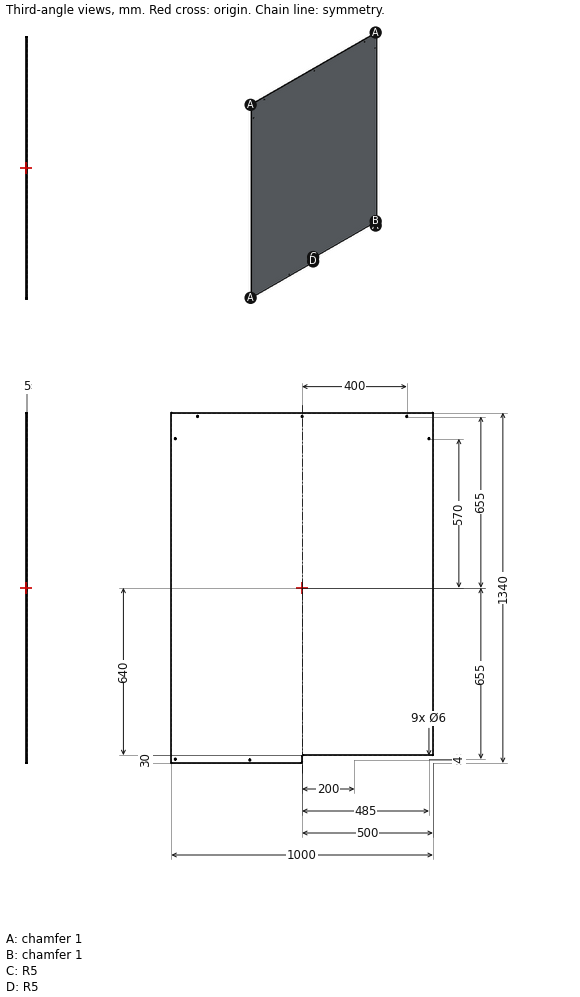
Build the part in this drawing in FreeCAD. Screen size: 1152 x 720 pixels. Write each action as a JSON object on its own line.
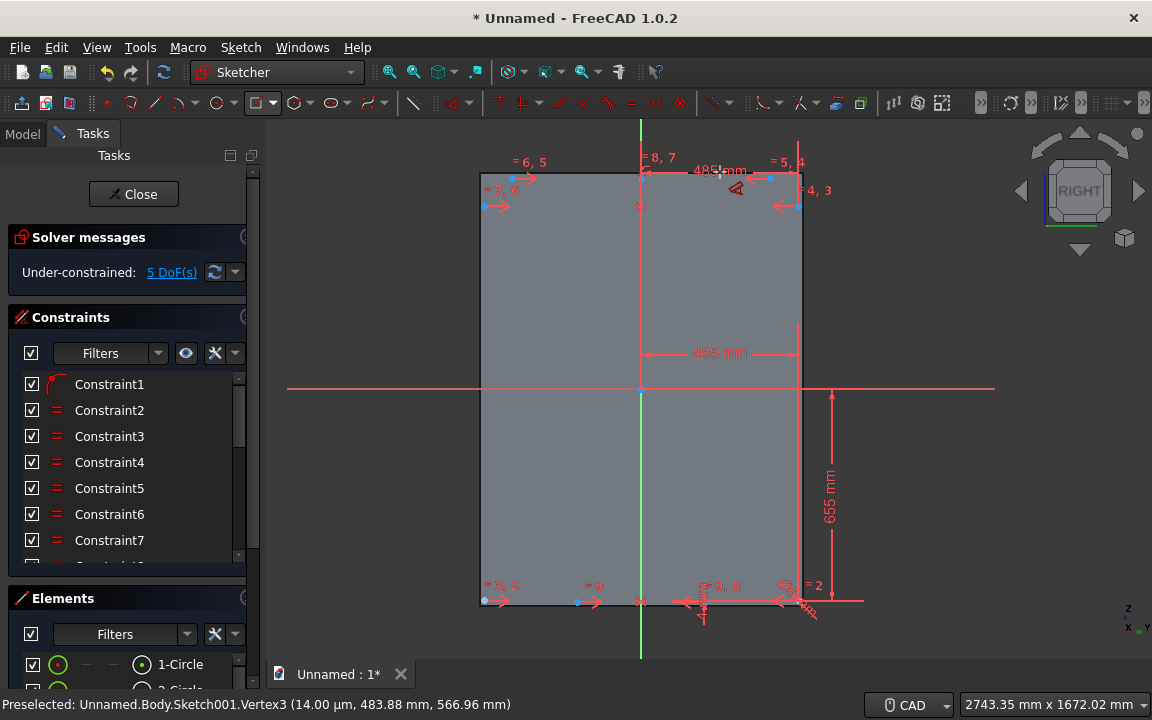
{"action": "left_click", "coordinate": [798, 206]}
{"action": "left_click", "coordinate": [832, 298]}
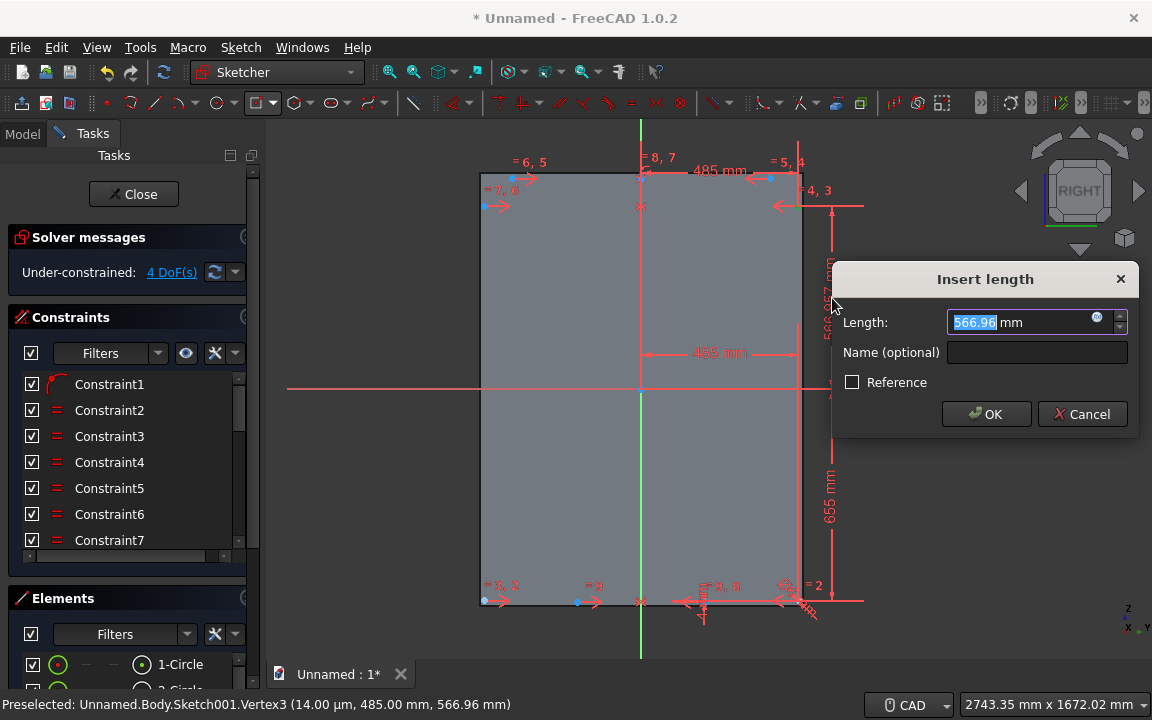
{"action": "type", "text": "570"}
{"action": "key", "text": "Return"}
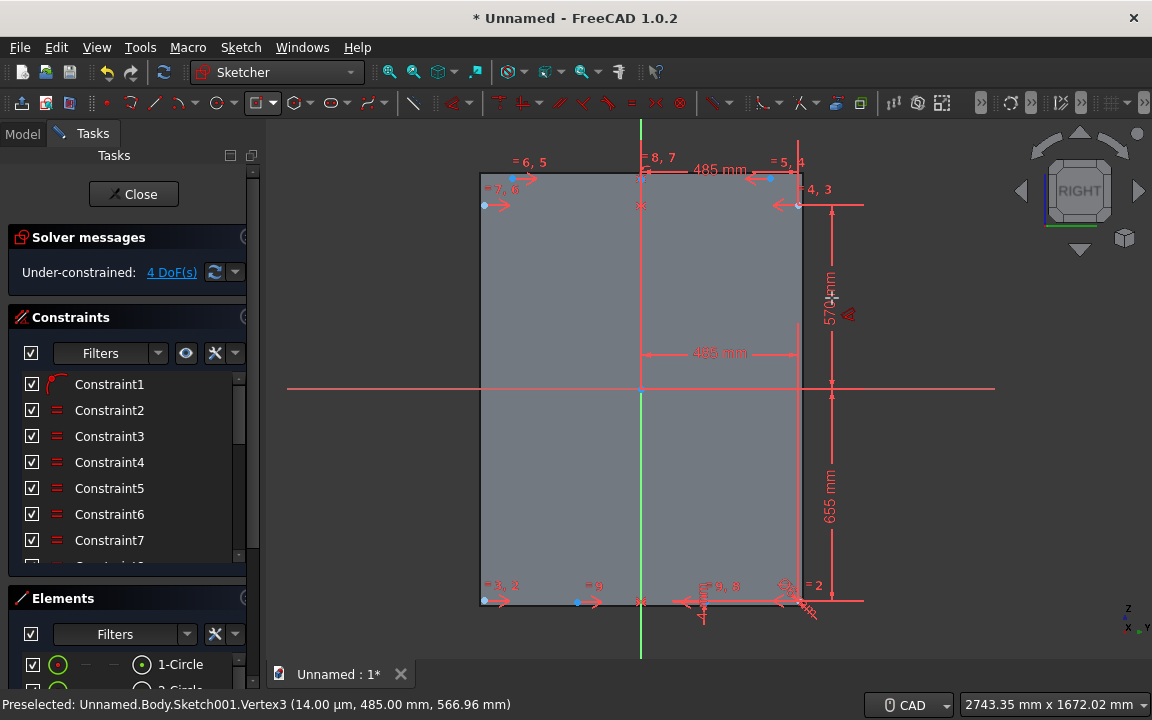
{"action": "left_click", "coordinate": [771, 179]}
{"action": "left_click", "coordinate": [706, 423]}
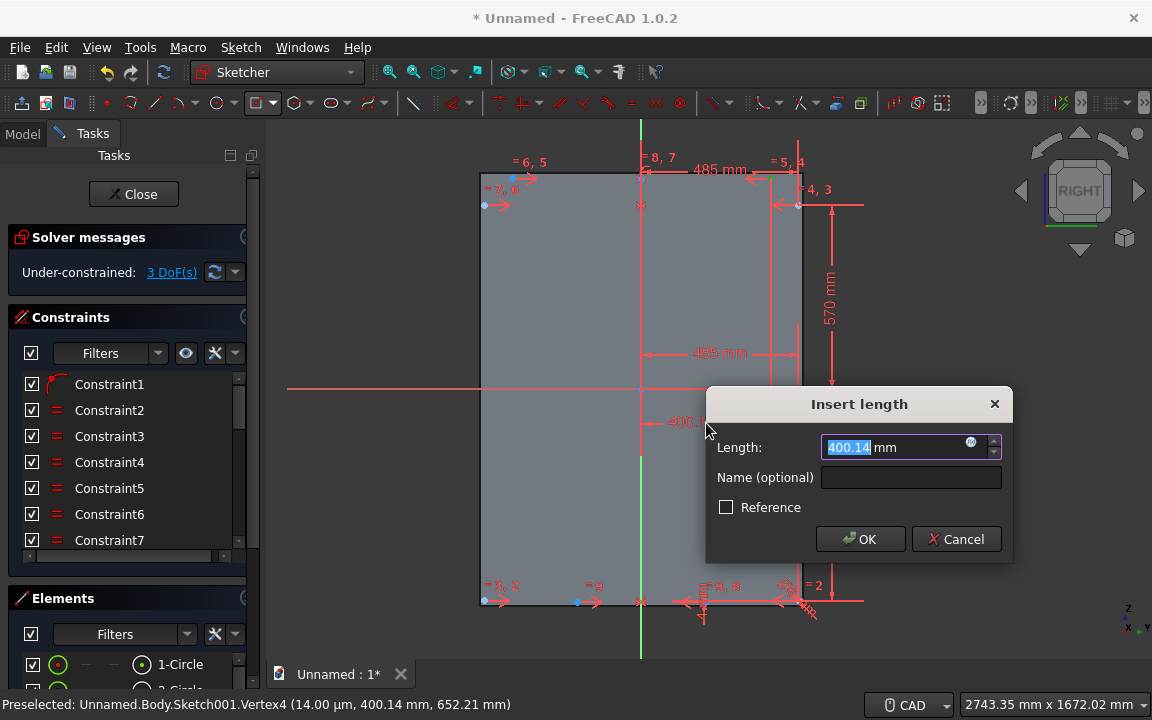
{"action": "type", "text": "400"}
{"action": "key", "text": "Return"}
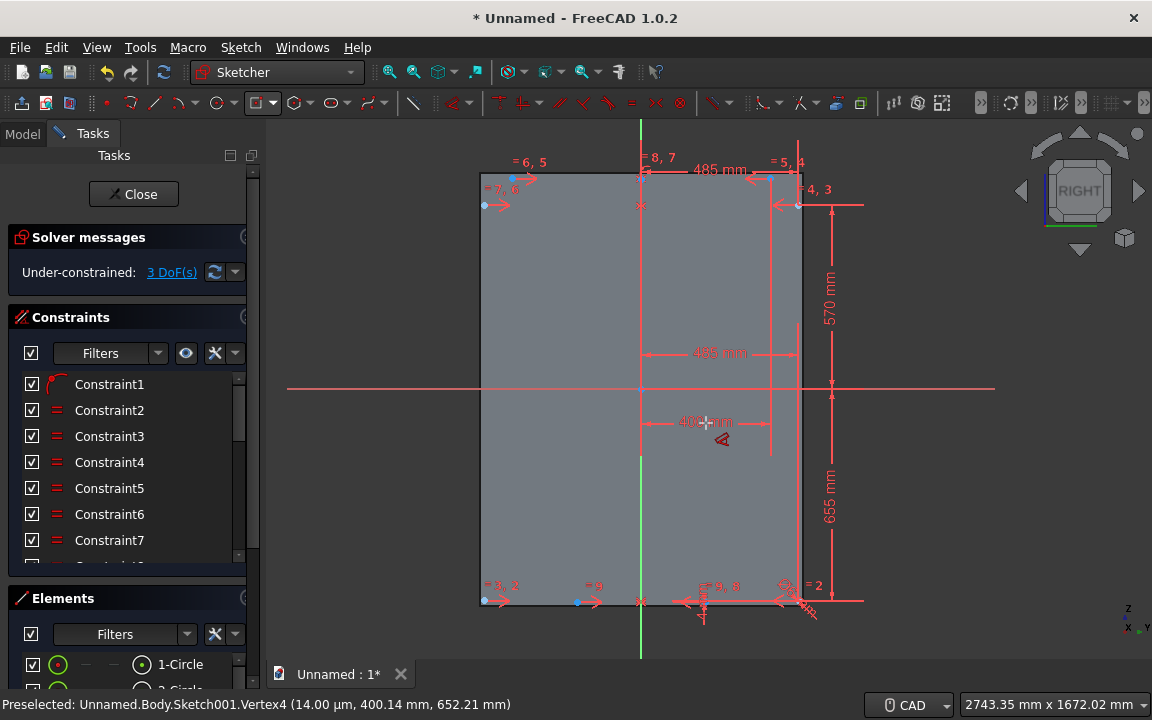
{"action": "left_click", "coordinate": [771, 179]}
{"action": "left_click", "coordinate": [805, 236]}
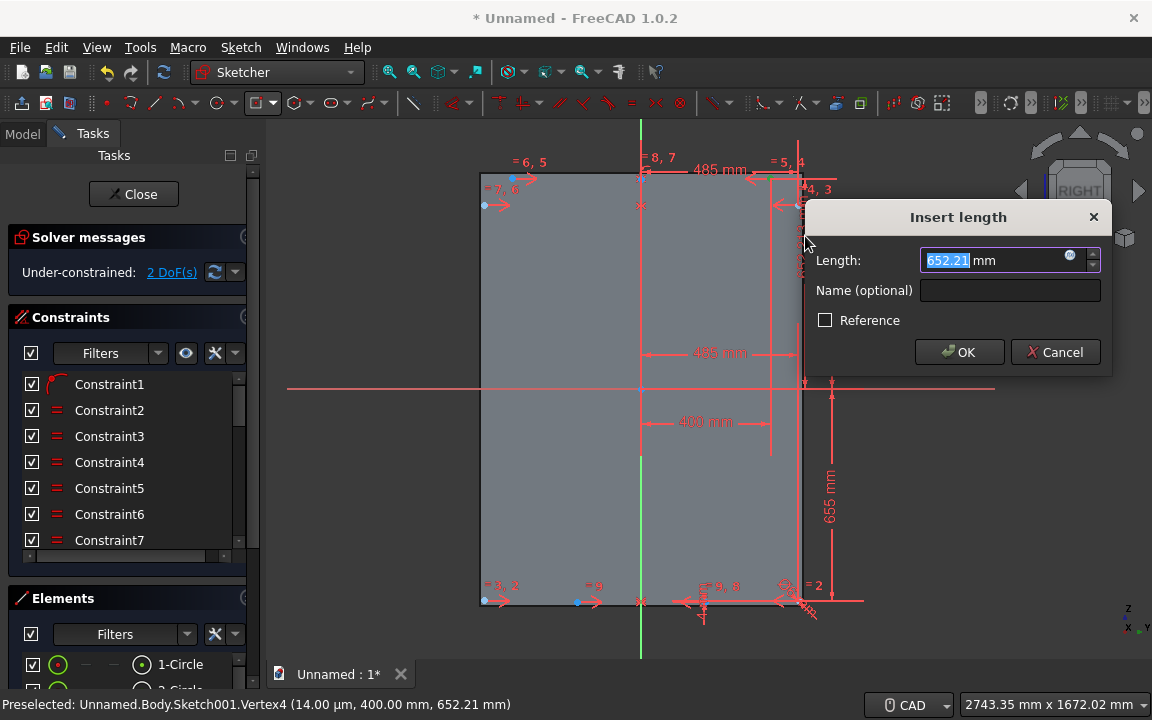
{"action": "type", "text": "655"}
{"action": "key", "text": "Return"}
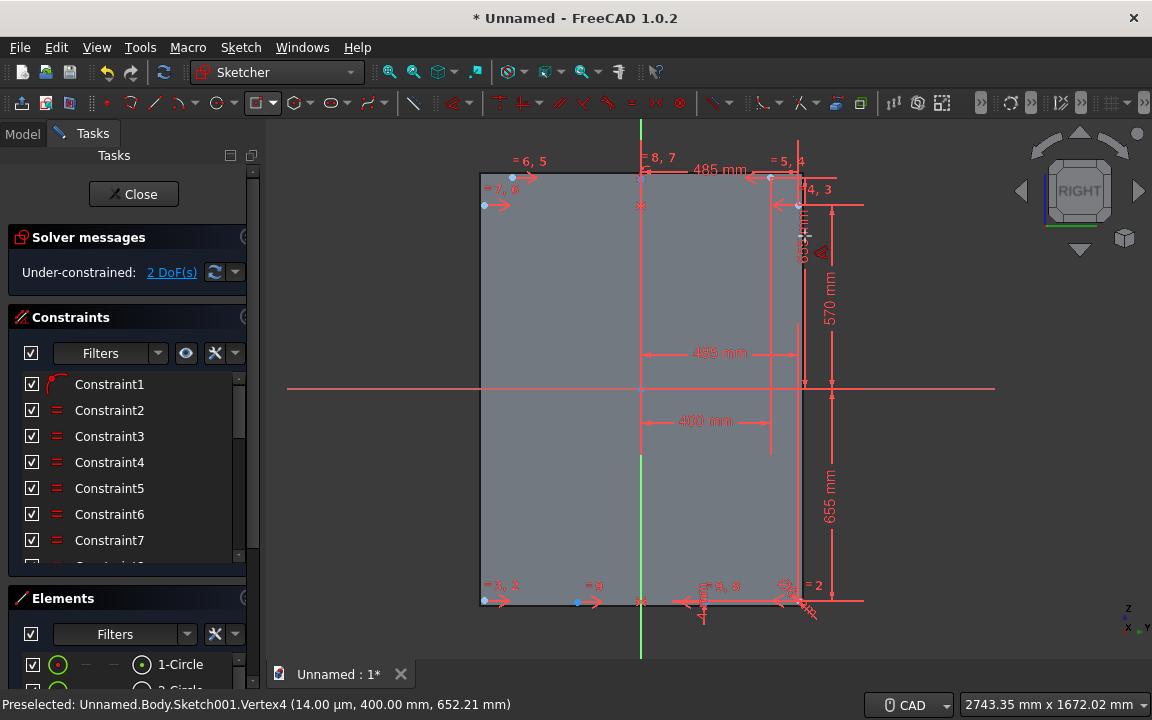
{"action": "left_click", "coordinate": [641, 179]}
{"action": "left_click", "coordinate": [675, 284]}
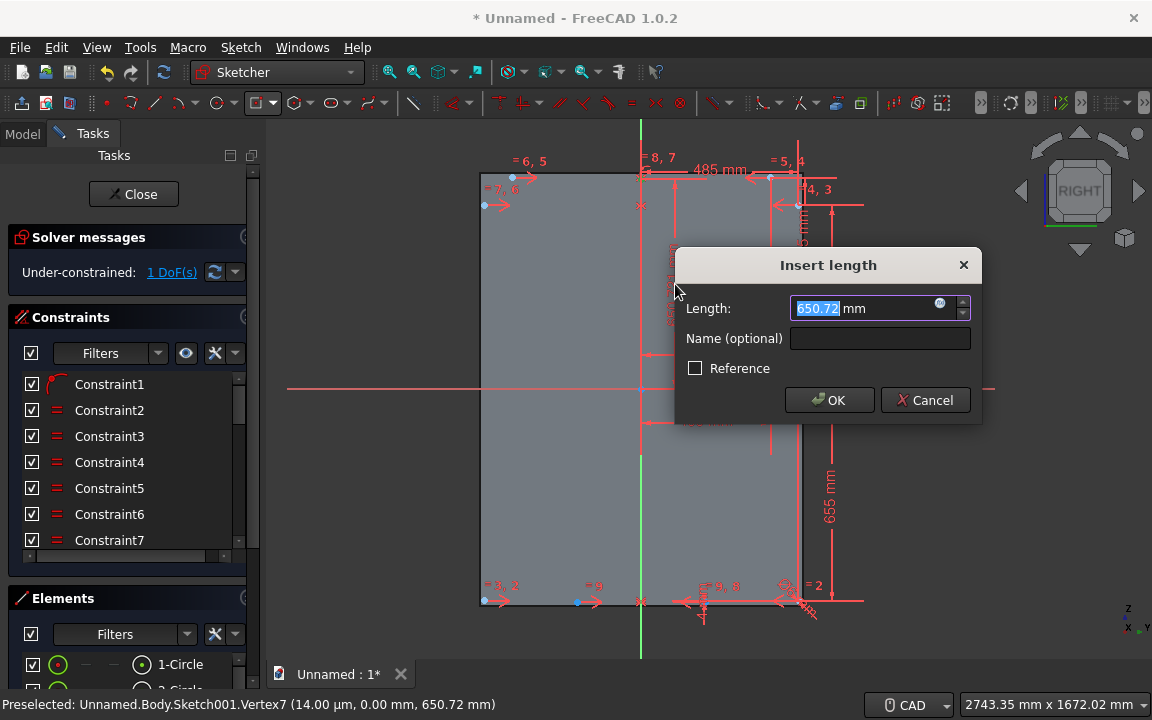
{"action": "type", "text": "655"}
{"action": "key", "text": "Return"}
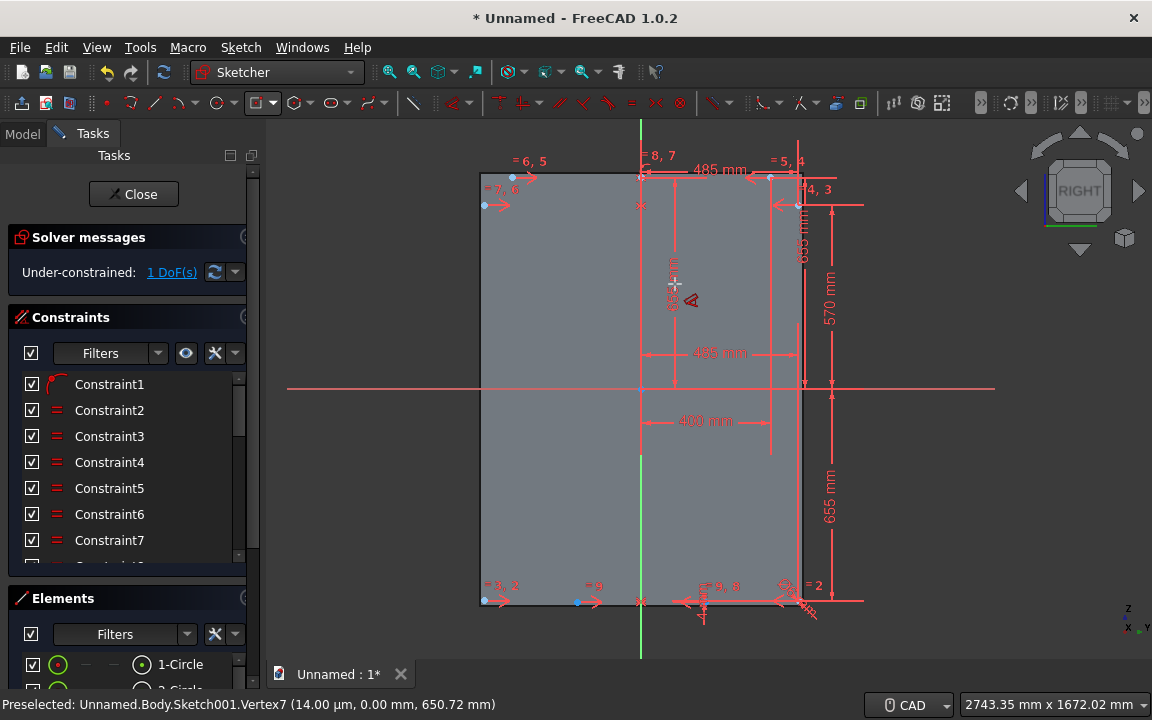
{"action": "left_click", "coordinate": [706, 602]}
{"action": "left_click", "coordinate": [674, 331]}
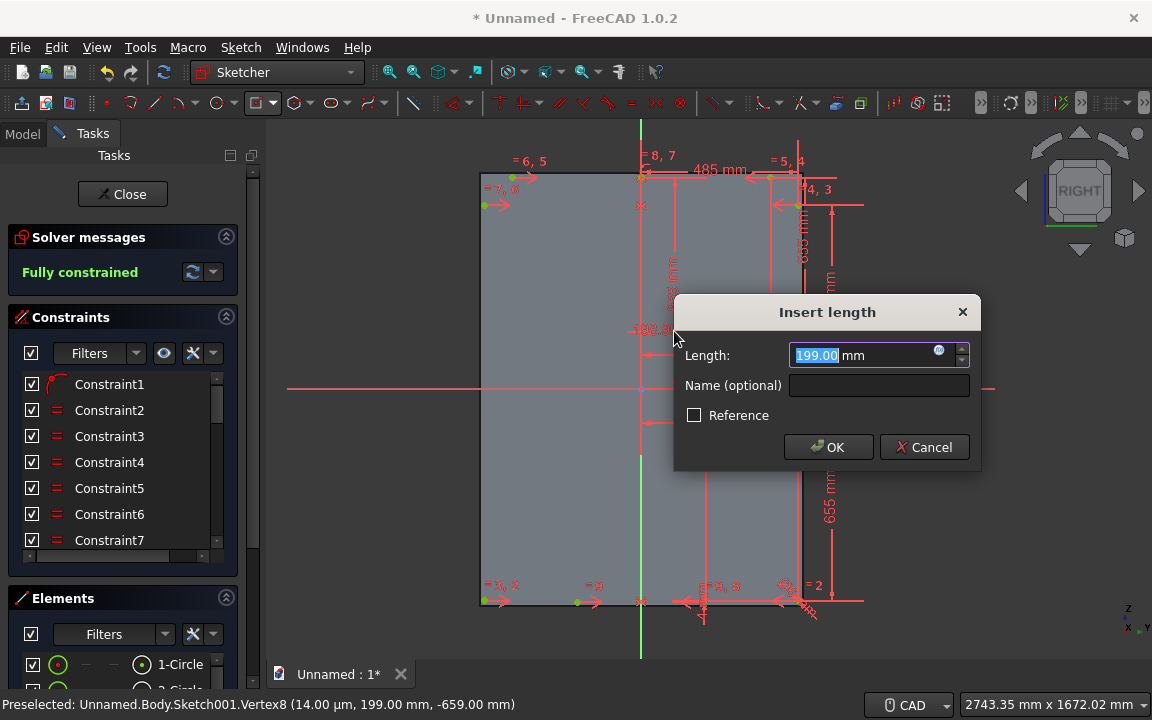
{"action": "type", "text": "200"}
{"action": "key", "text": "Return"}
{"action": "key", "text": "Escape"}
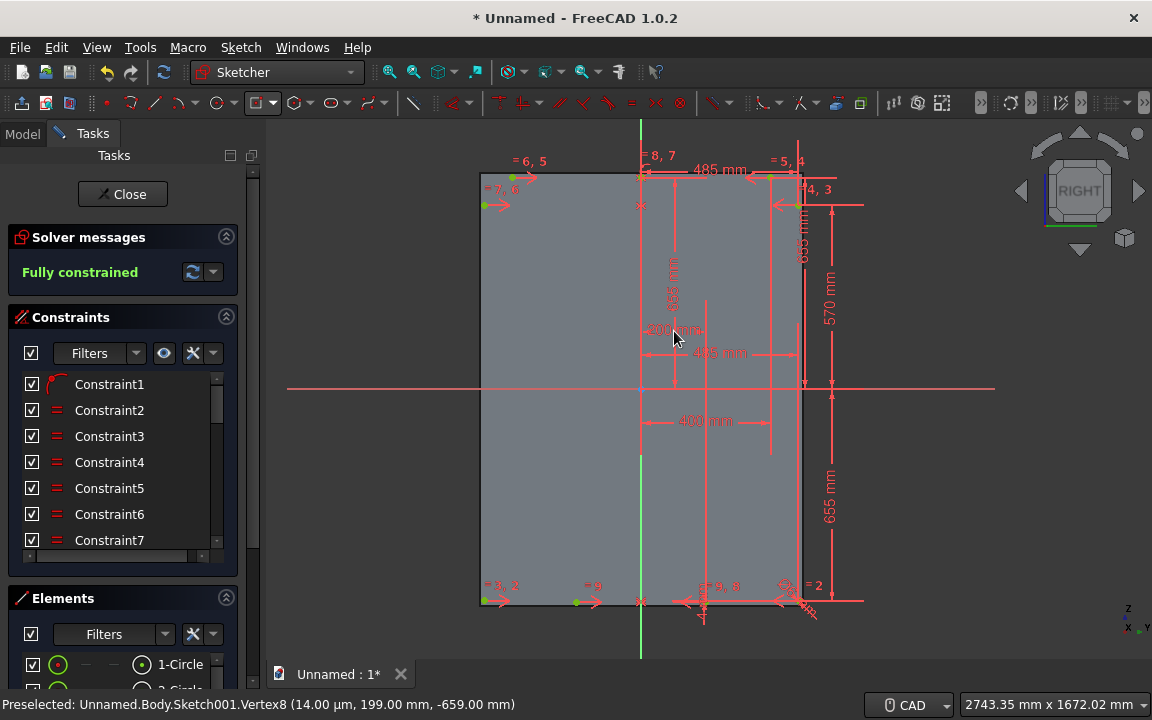
{"action": "left_click", "coordinate": [123, 194]}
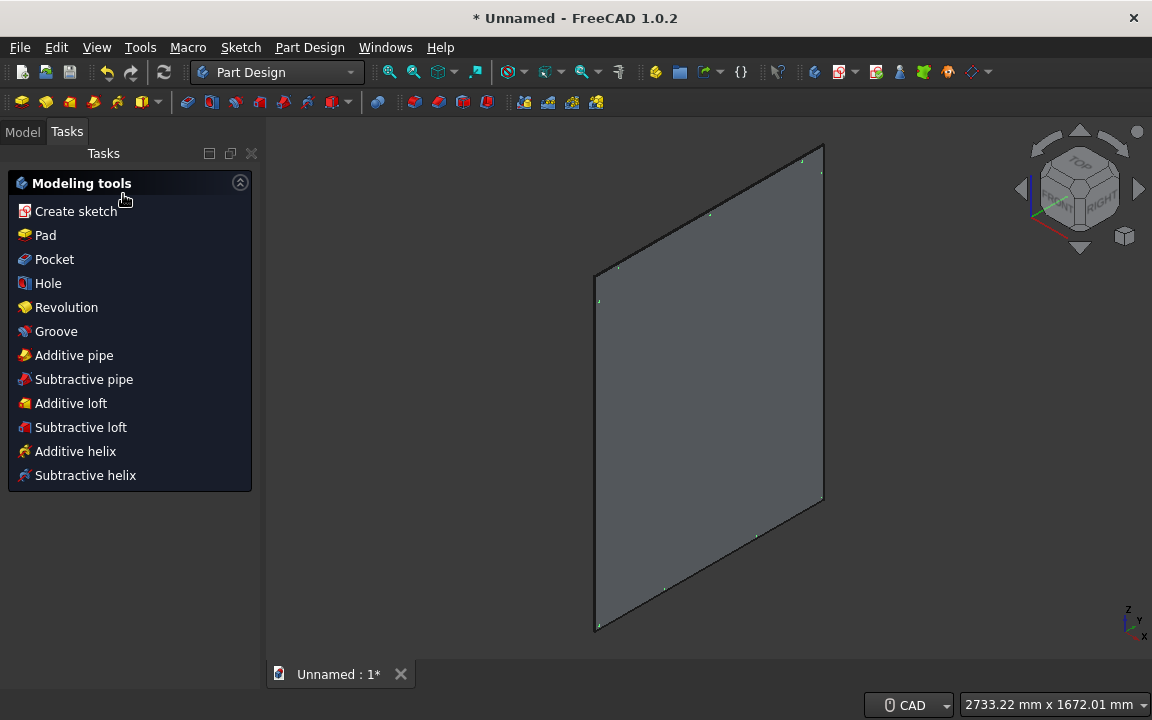
{"action": "left_click", "coordinate": [188, 102]}